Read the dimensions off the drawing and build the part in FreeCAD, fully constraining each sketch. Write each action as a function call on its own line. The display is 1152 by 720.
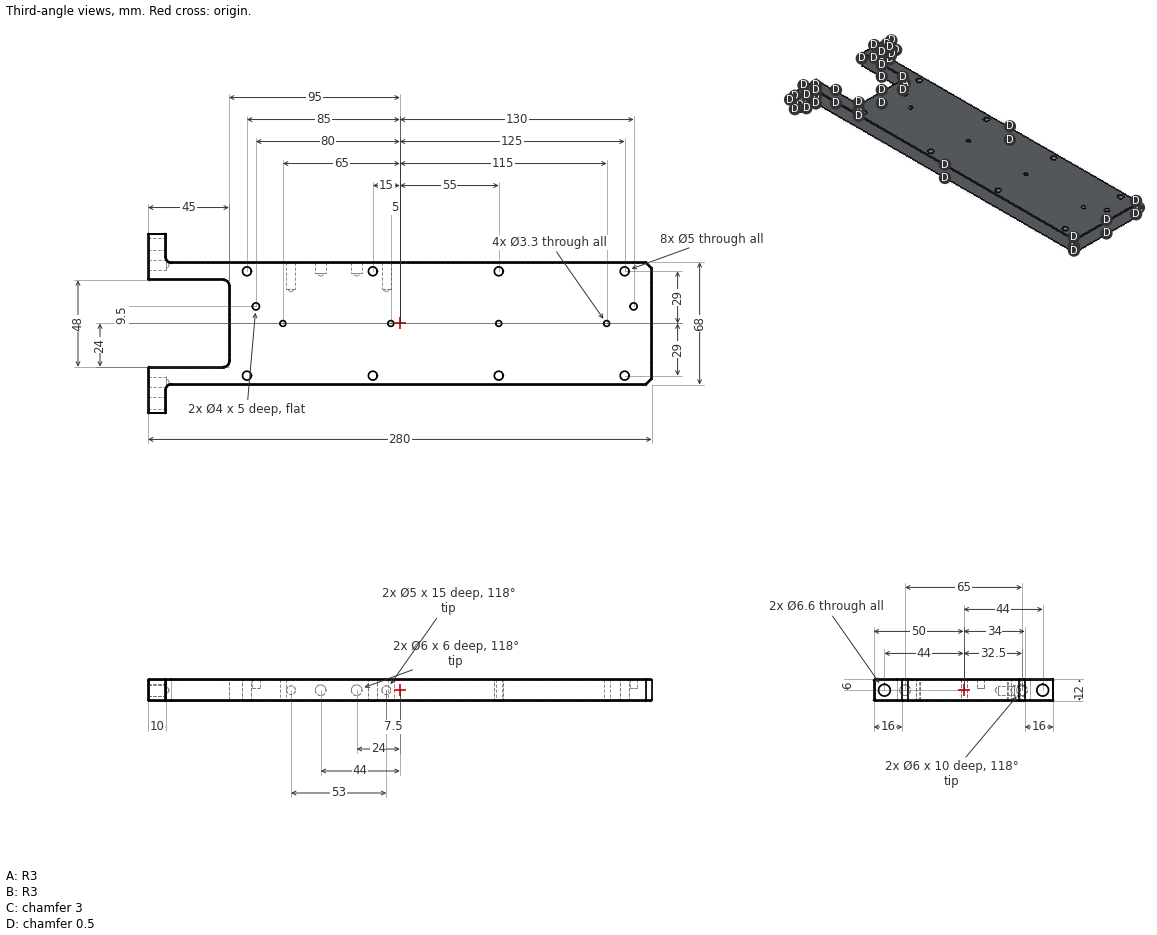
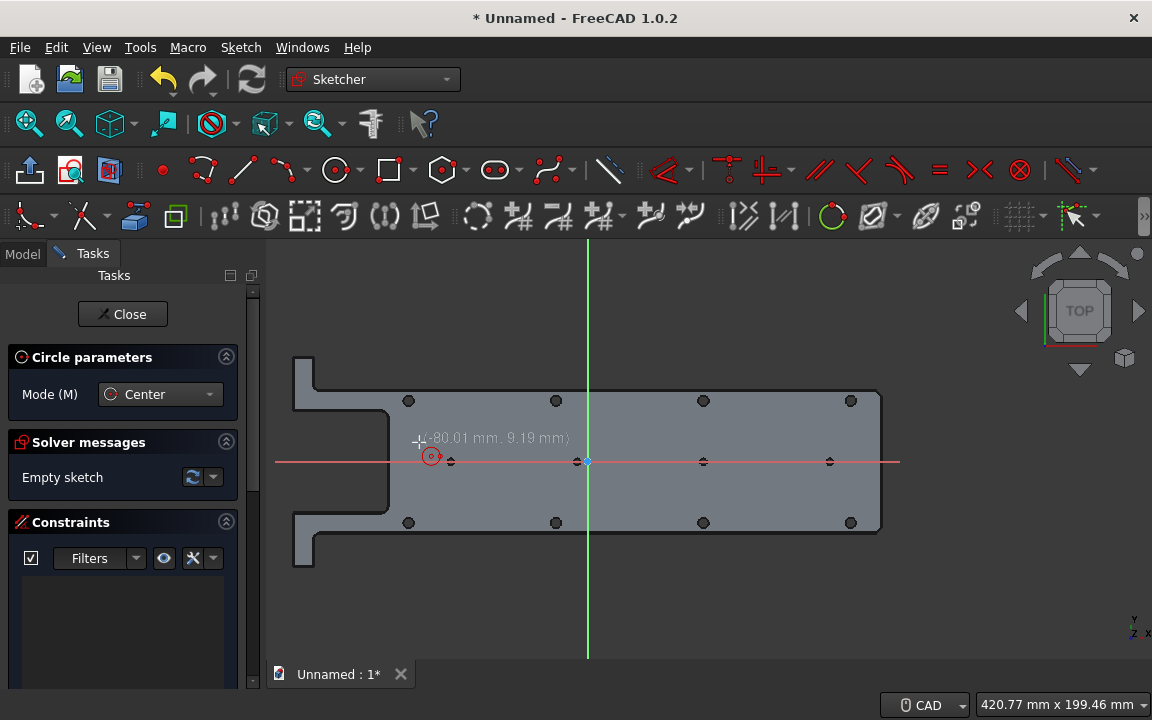
click(419, 442)
move(422, 439)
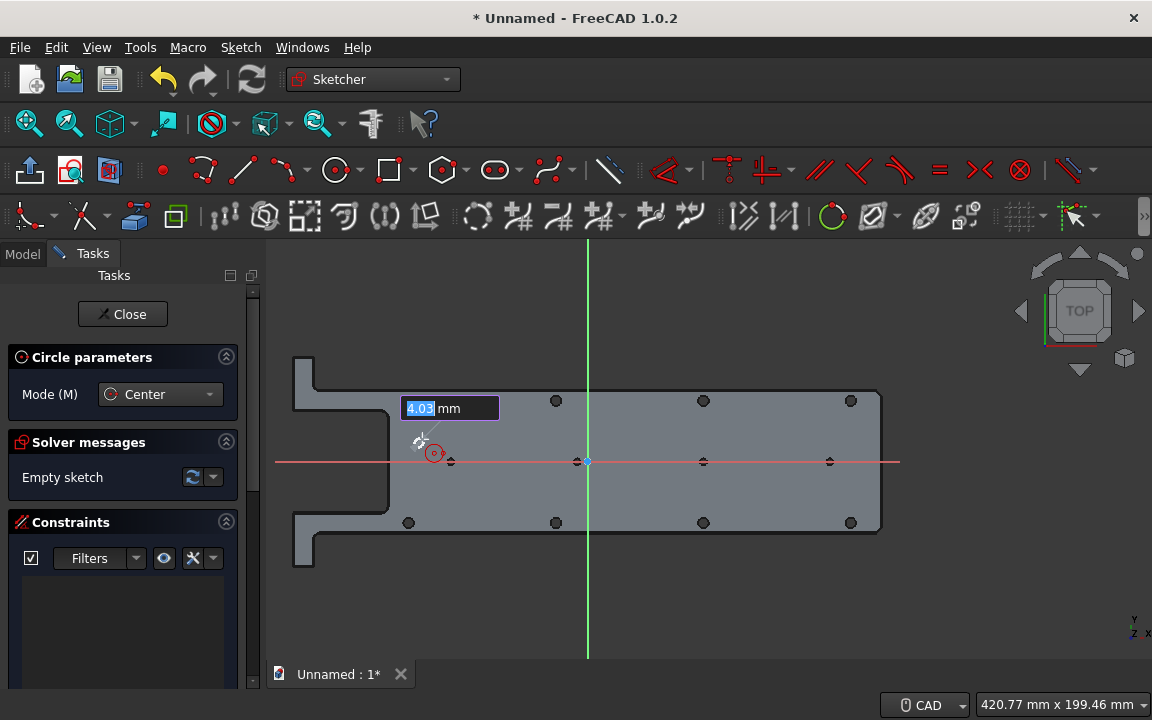
text(4)
key(Return)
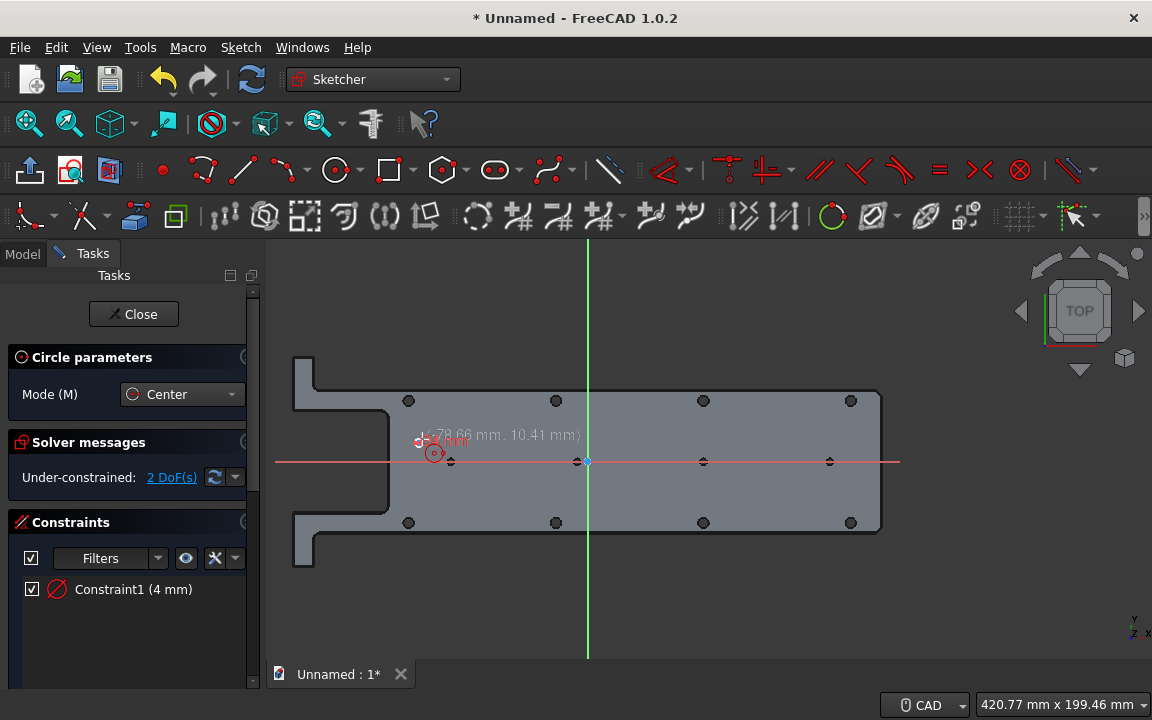
scroll(861, 442, up, 9)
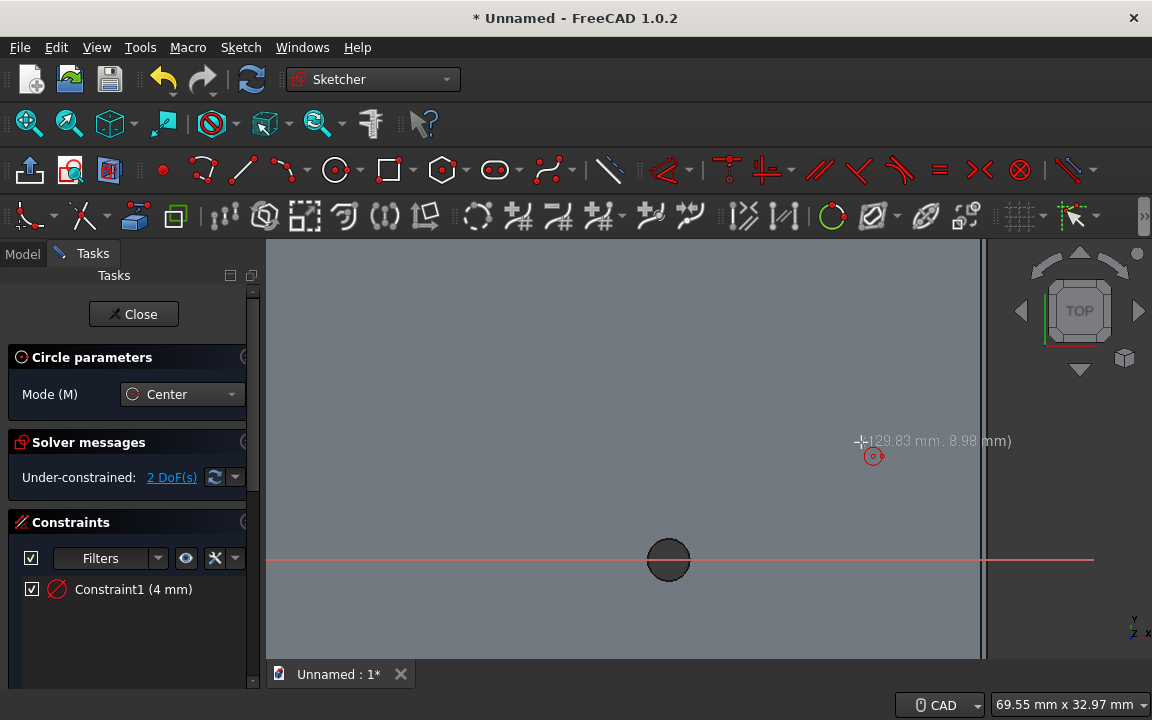
scroll(862, 442, down, 9)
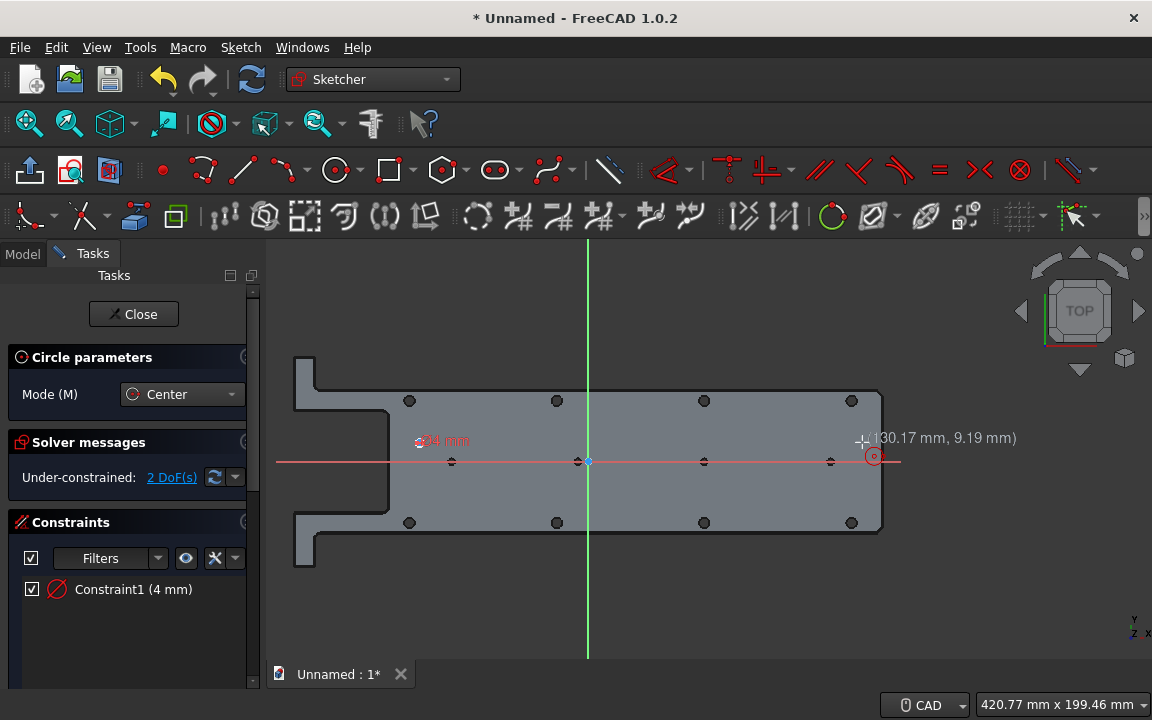
click(862, 442)
move(865, 439)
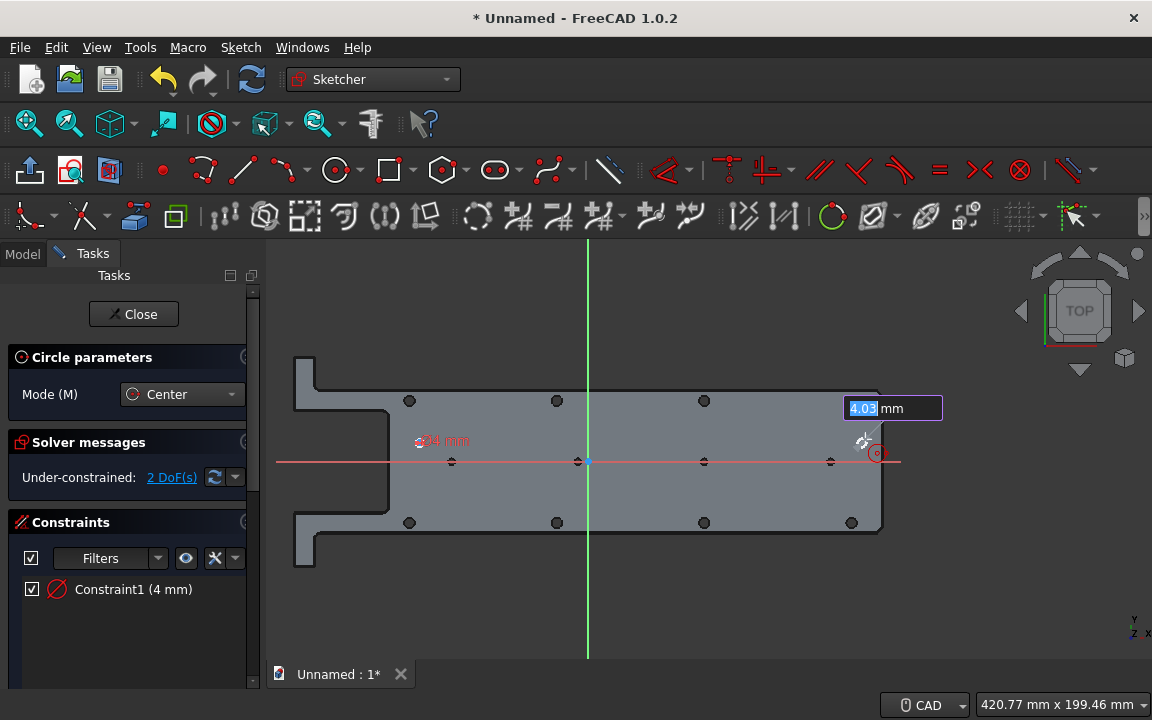
text(4)
key(Return)
key(Escape)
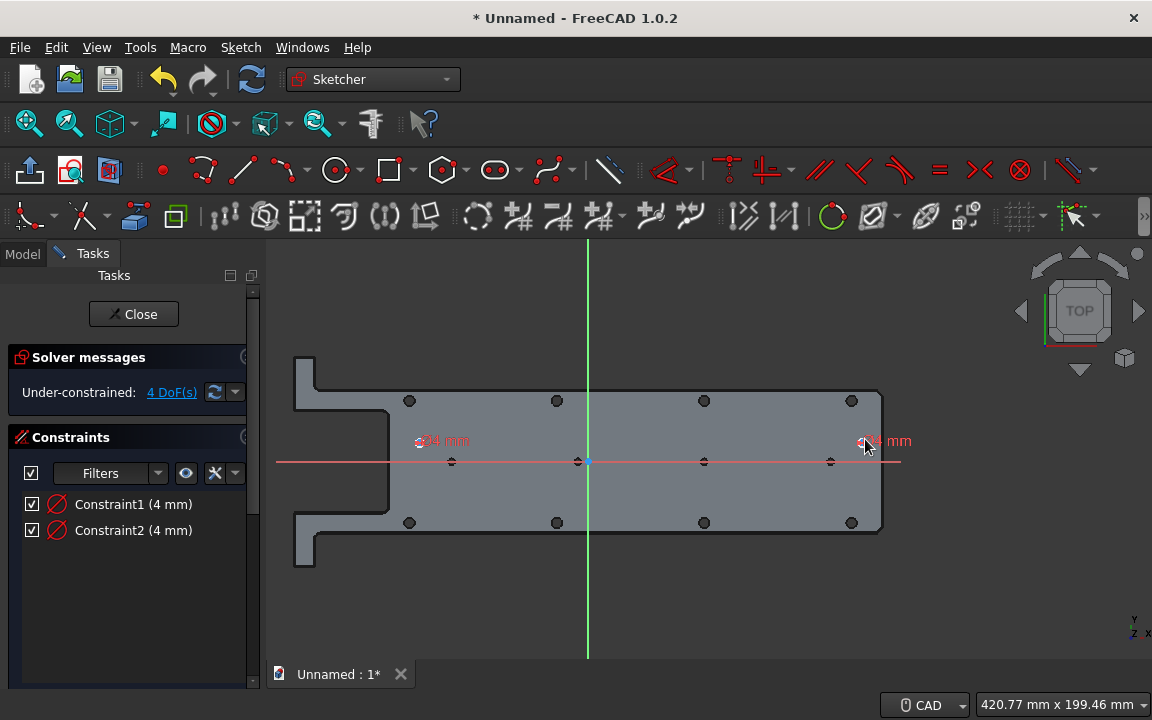
key(d)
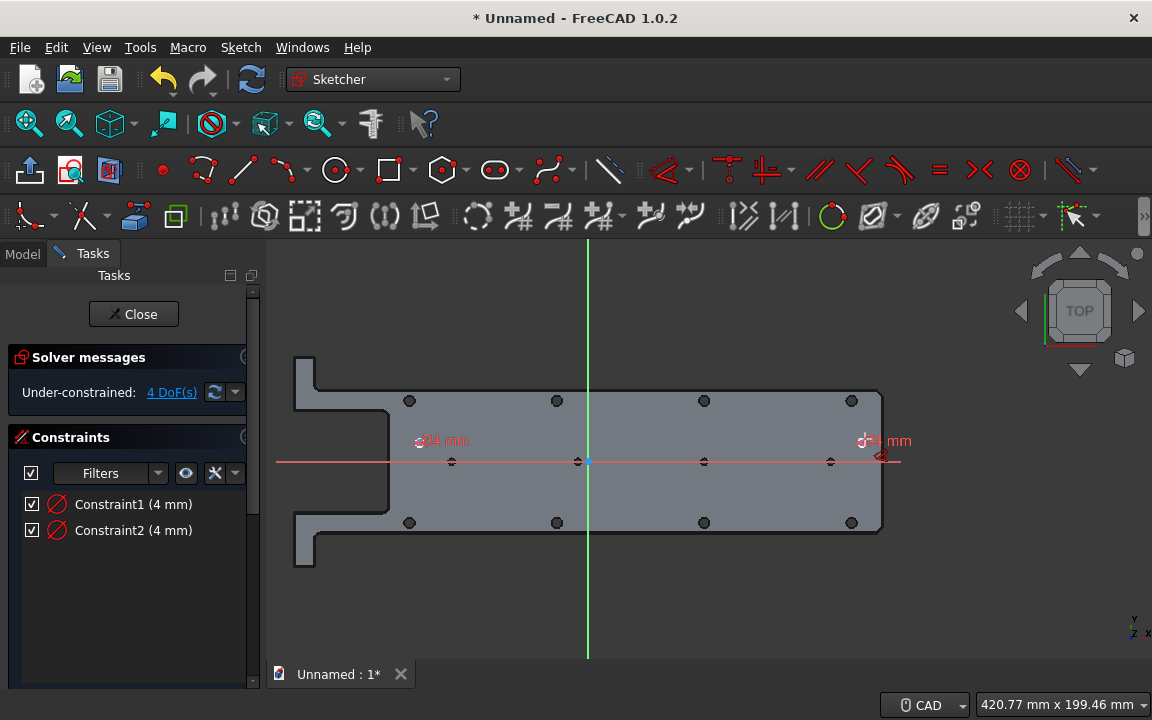
click(420, 443)
click(504, 496)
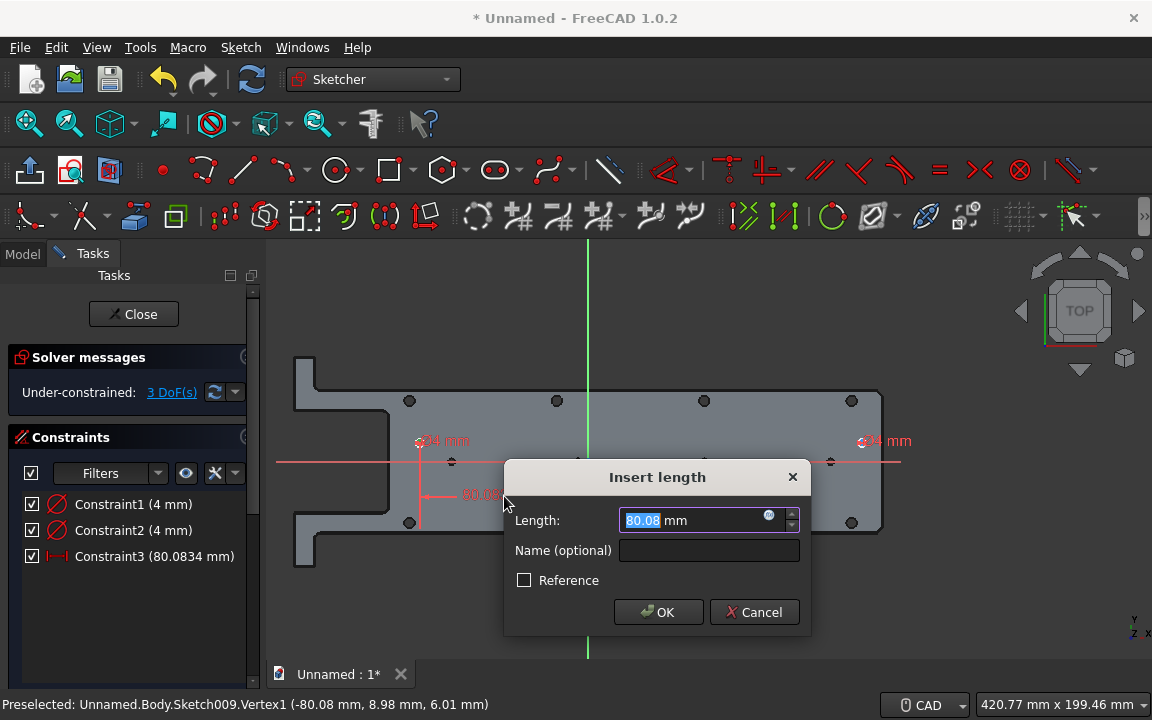
text(80)
key(Return)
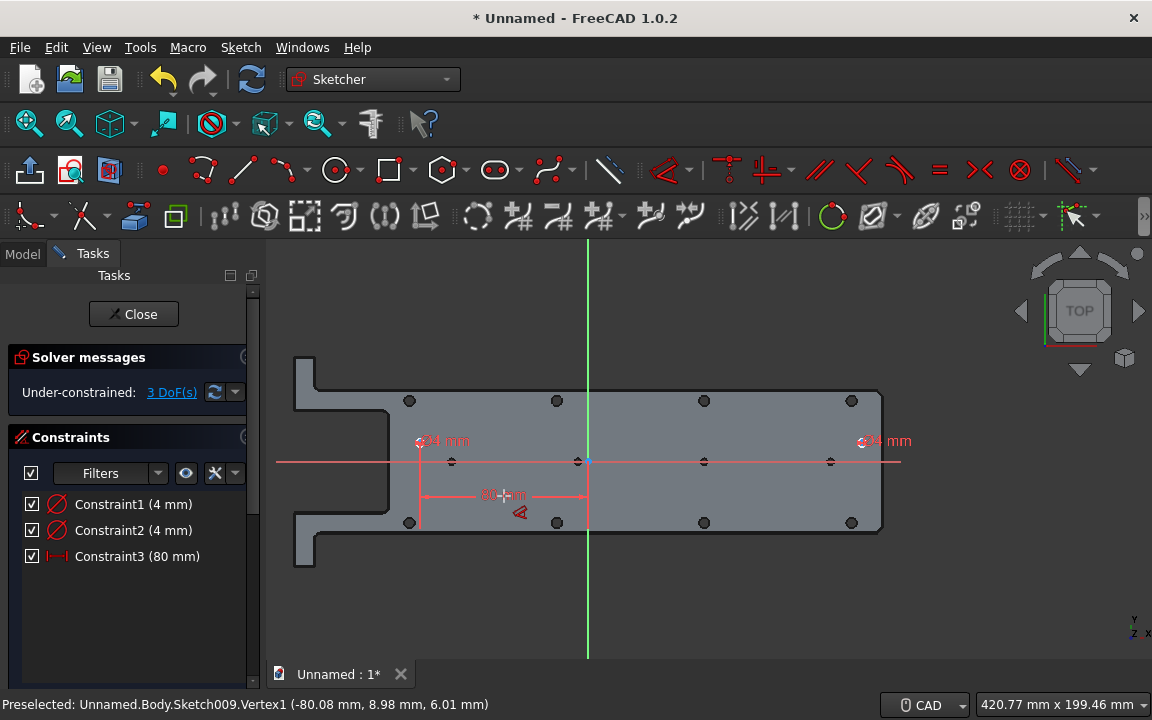
scroll(420, 443, up, 4)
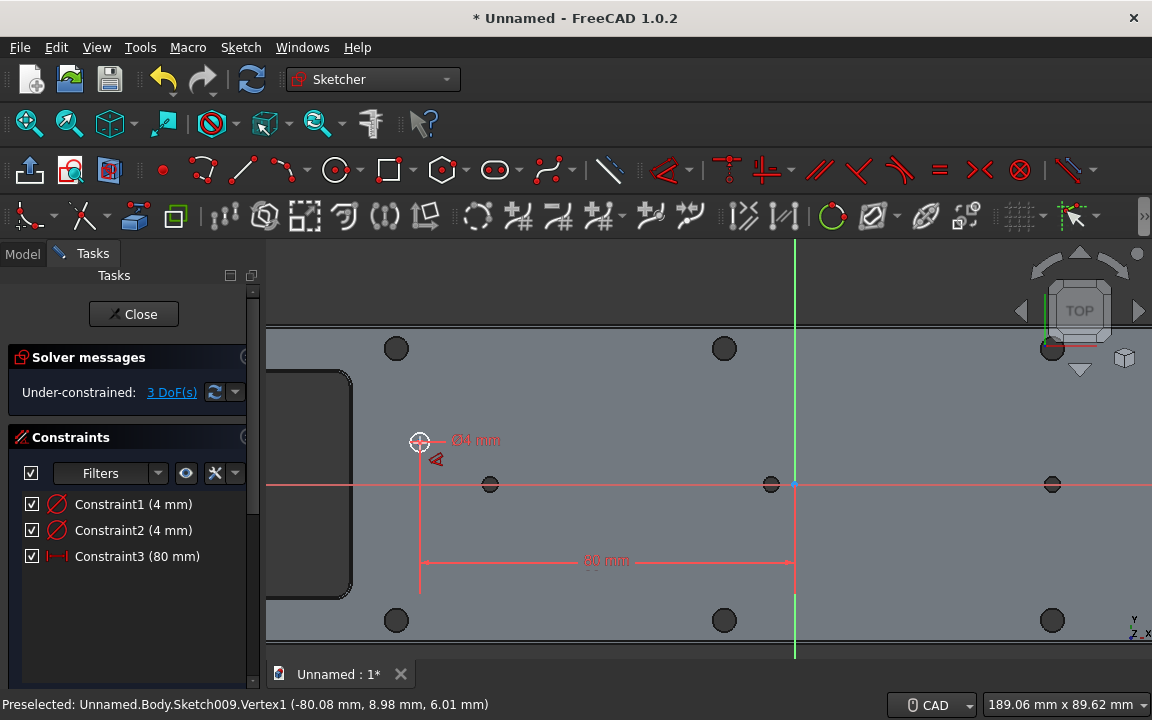
click(420, 442)
click(386, 463)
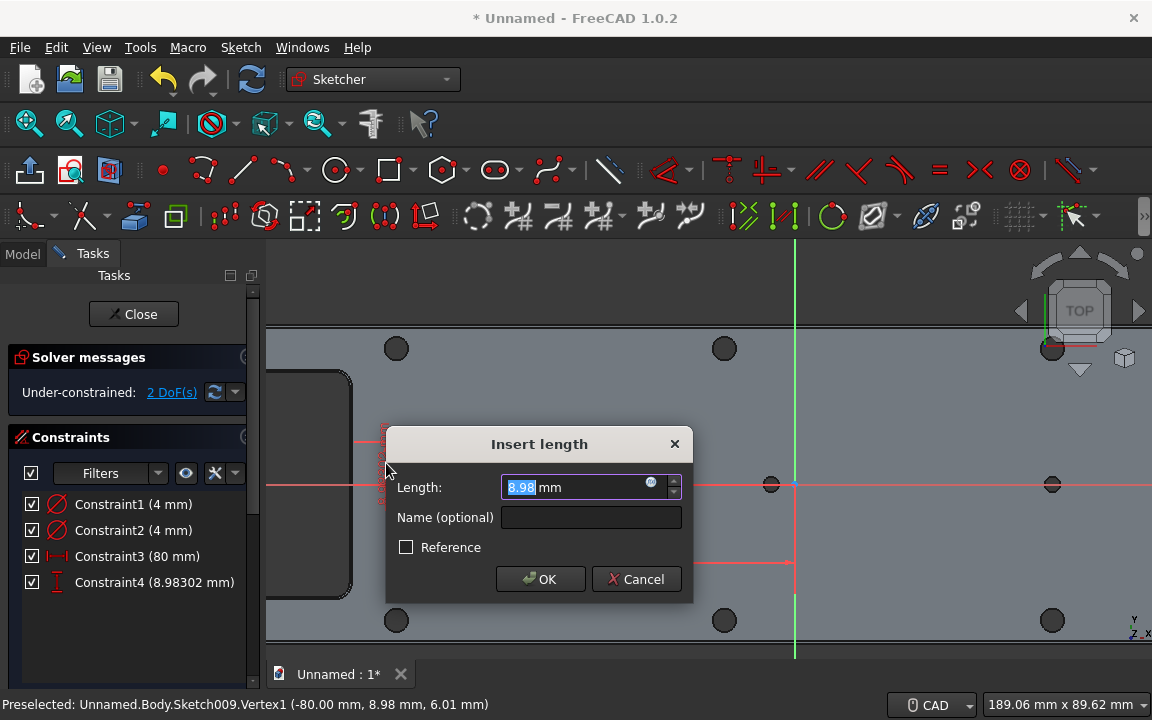
text(9.5)
key(Return)